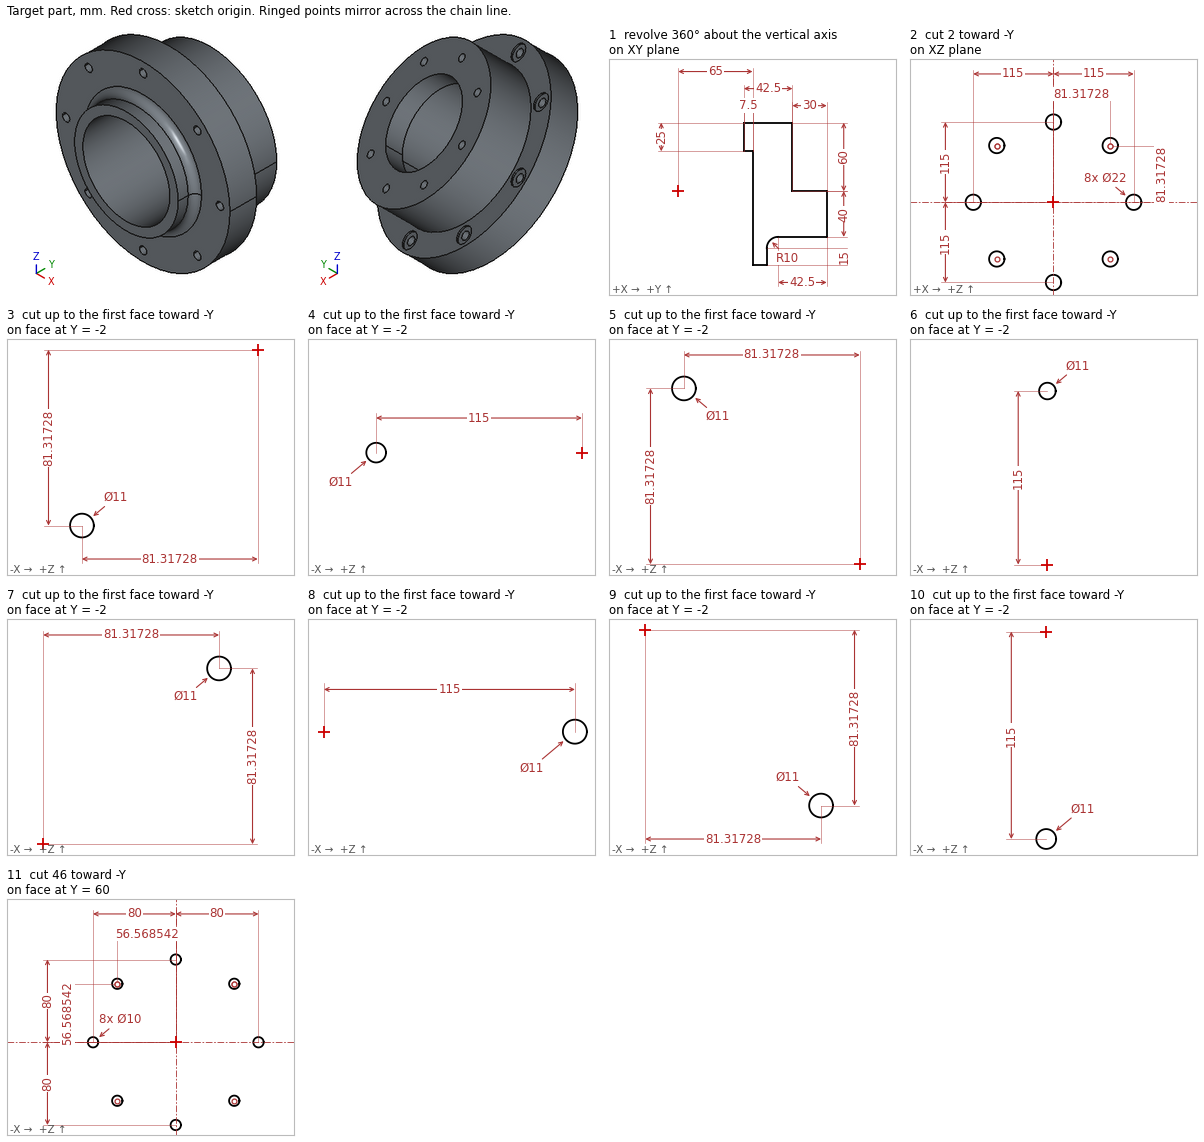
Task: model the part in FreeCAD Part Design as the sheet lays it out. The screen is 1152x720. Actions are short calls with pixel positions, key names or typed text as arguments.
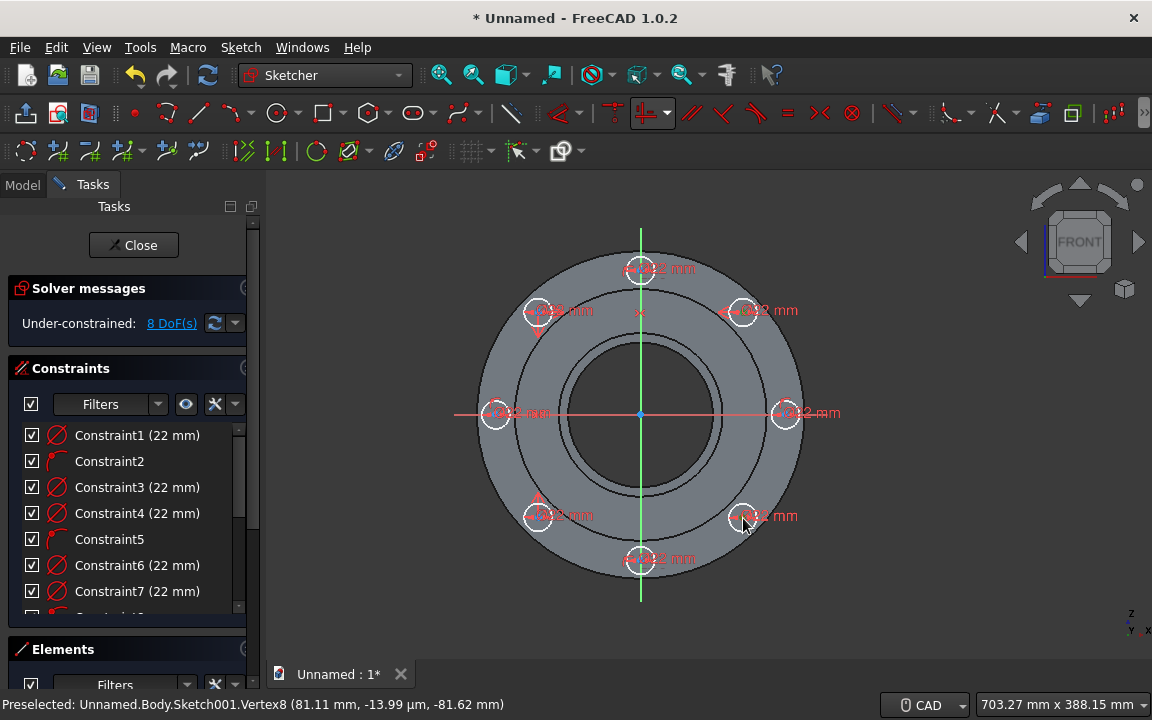
click(591, 415)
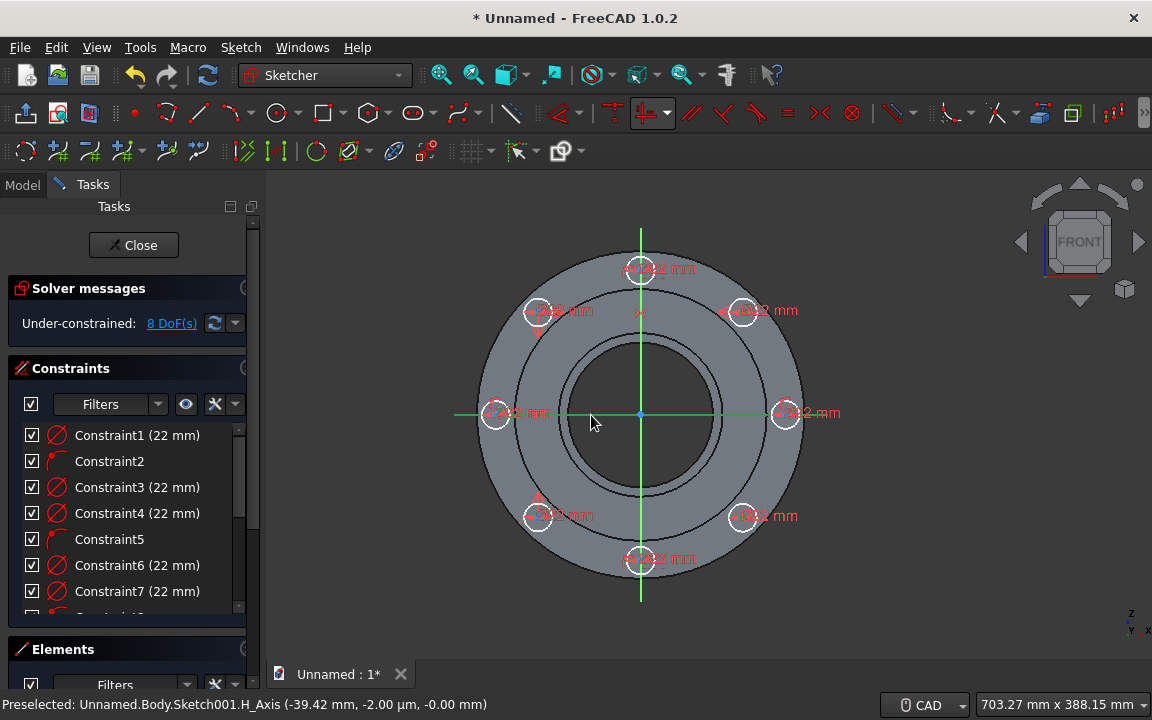
click(820, 114)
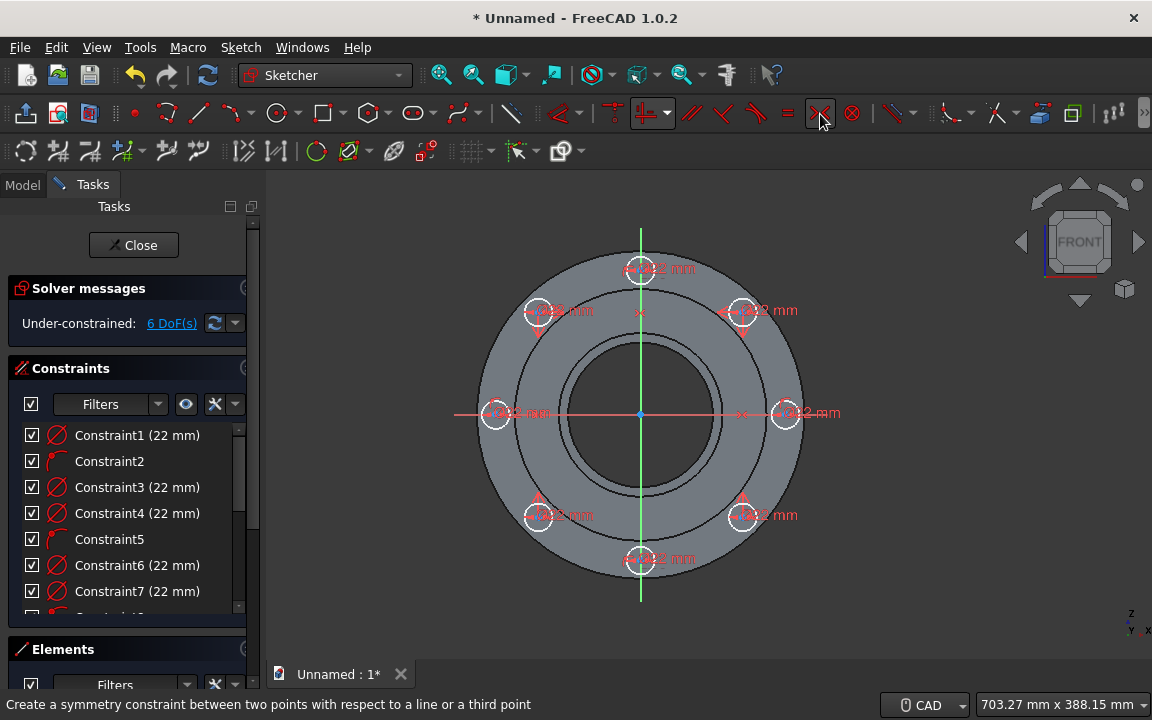
click(558, 114)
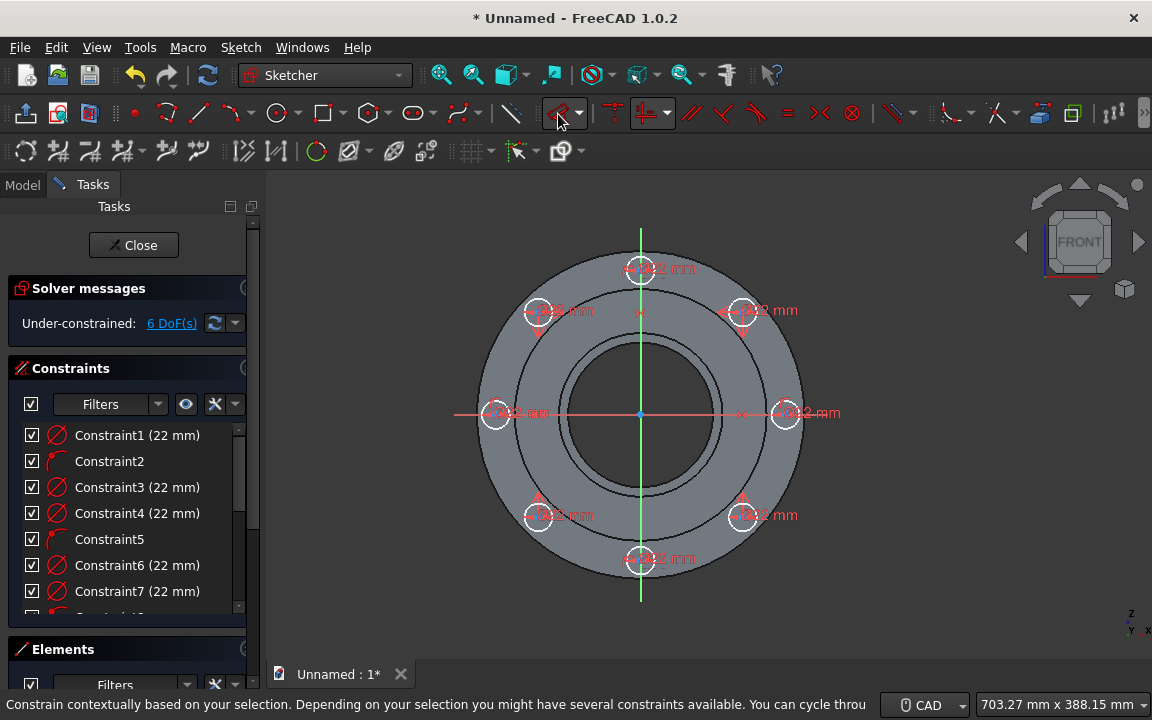
click(786, 415)
click(713, 449)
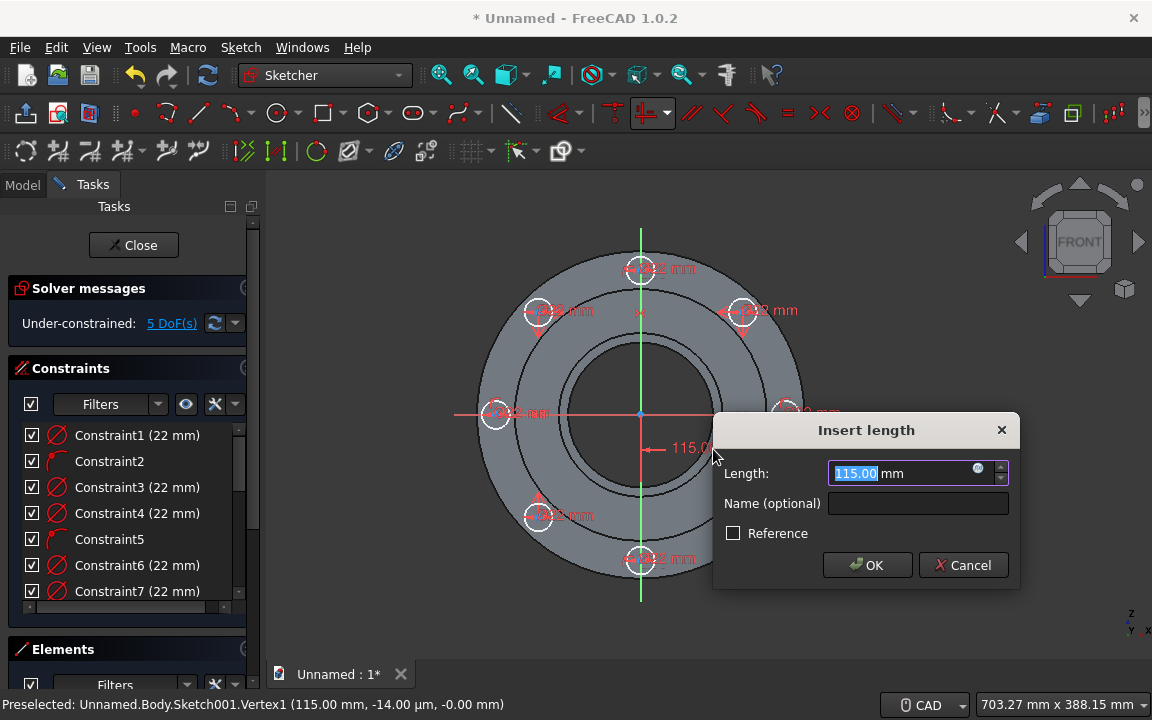
text(115)
key(Return)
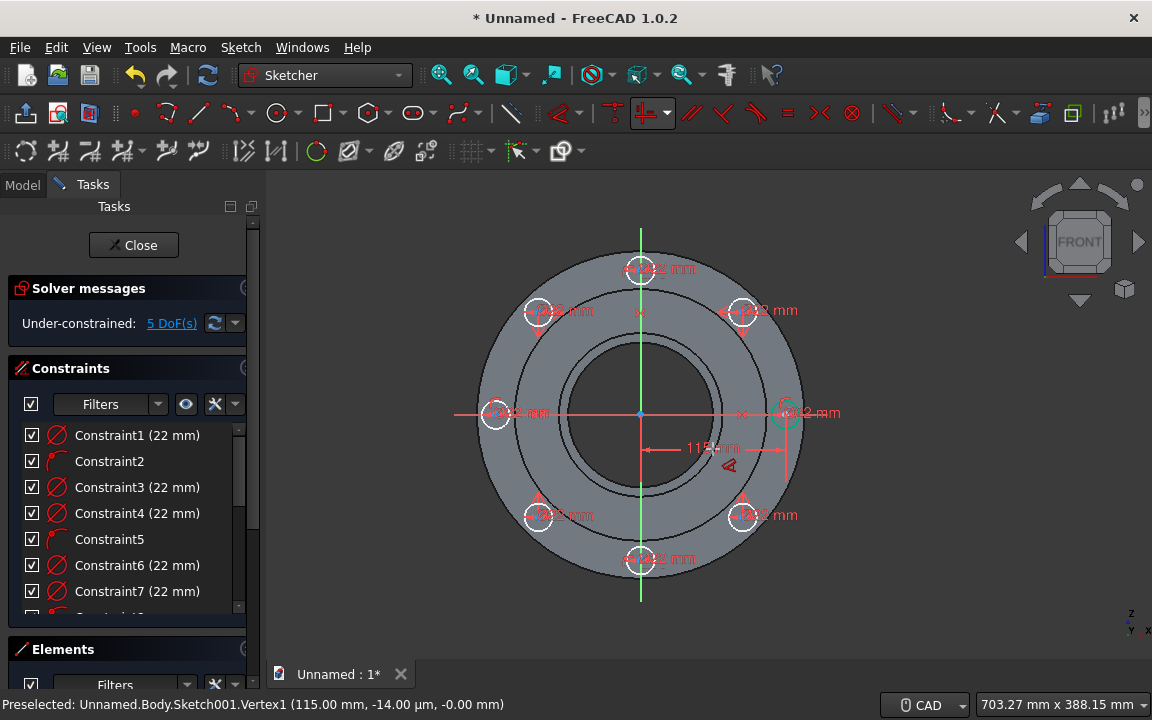
click(641, 271)
click(675, 343)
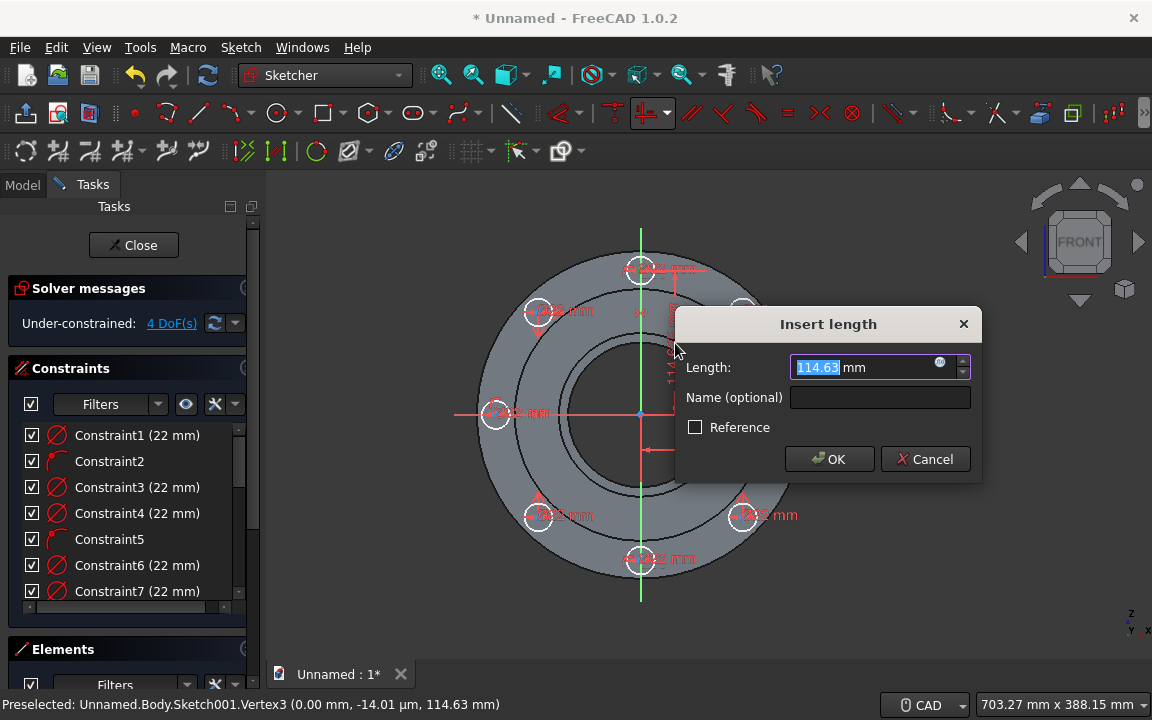
text(115)
key(Return)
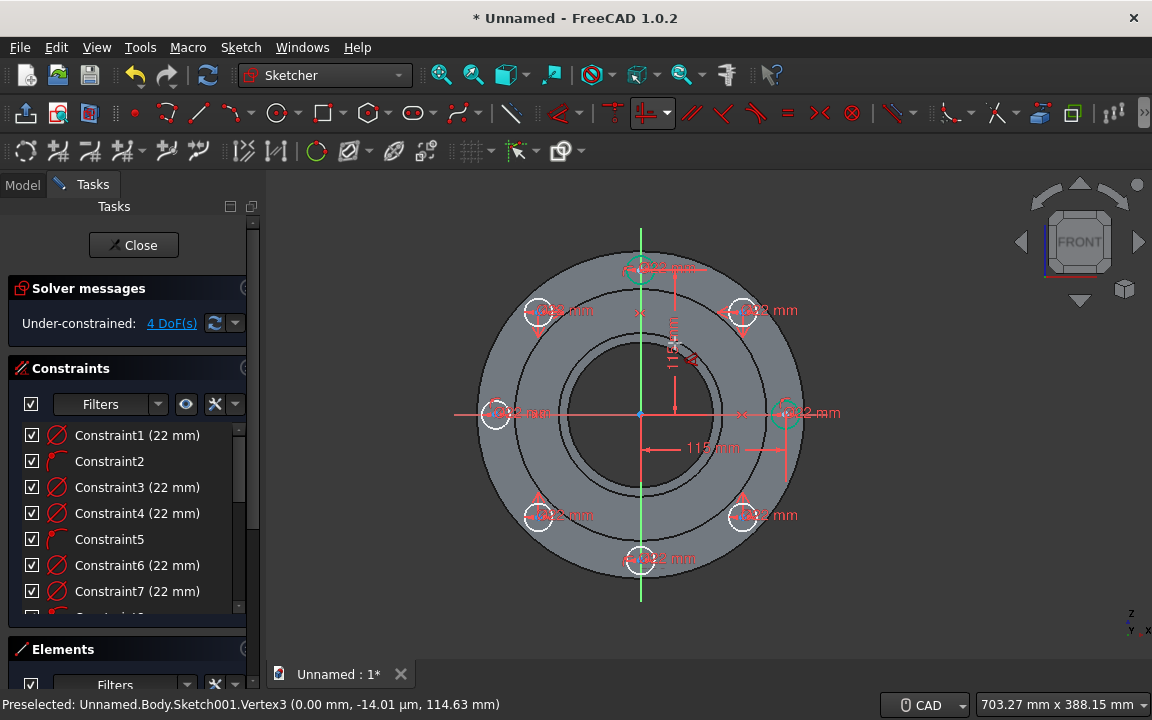
click(496, 415)
click(568, 449)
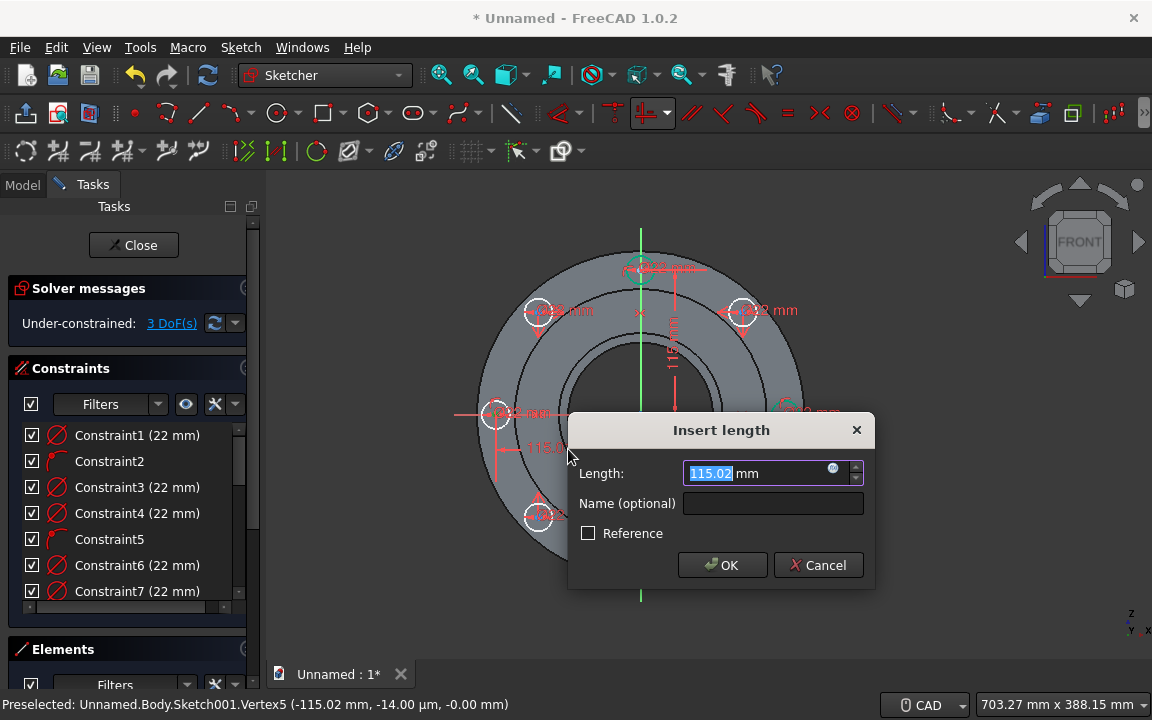
text(115)
key(Return)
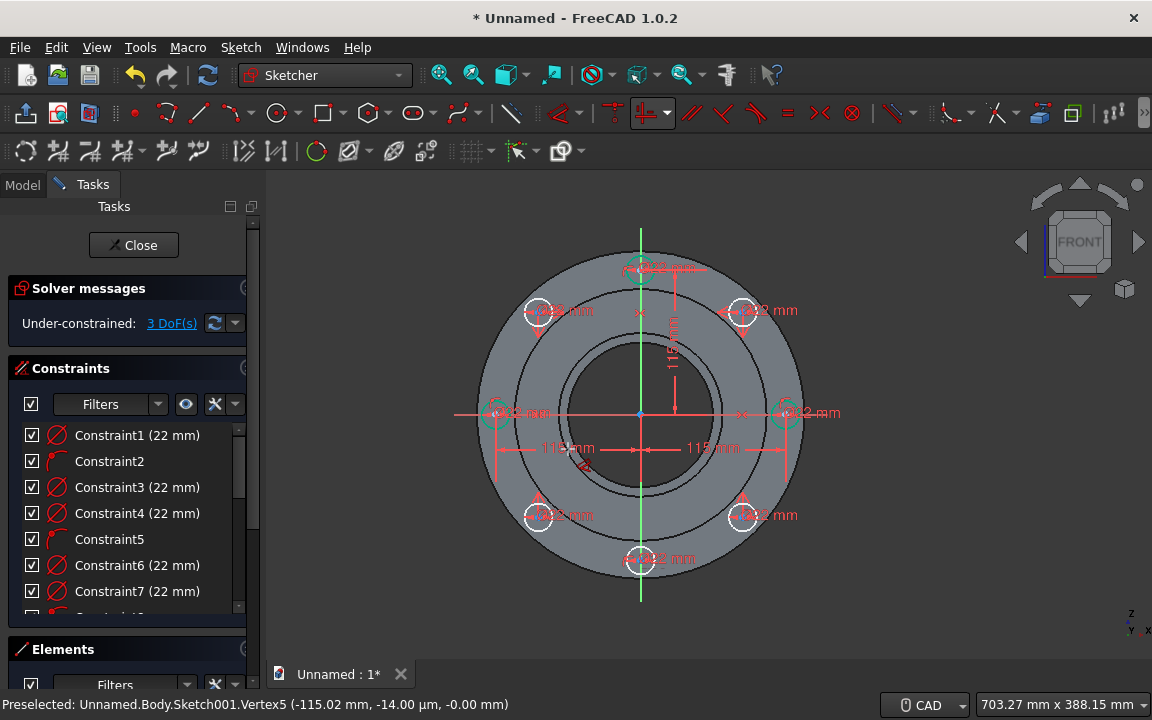
click(641, 561)
click(675, 488)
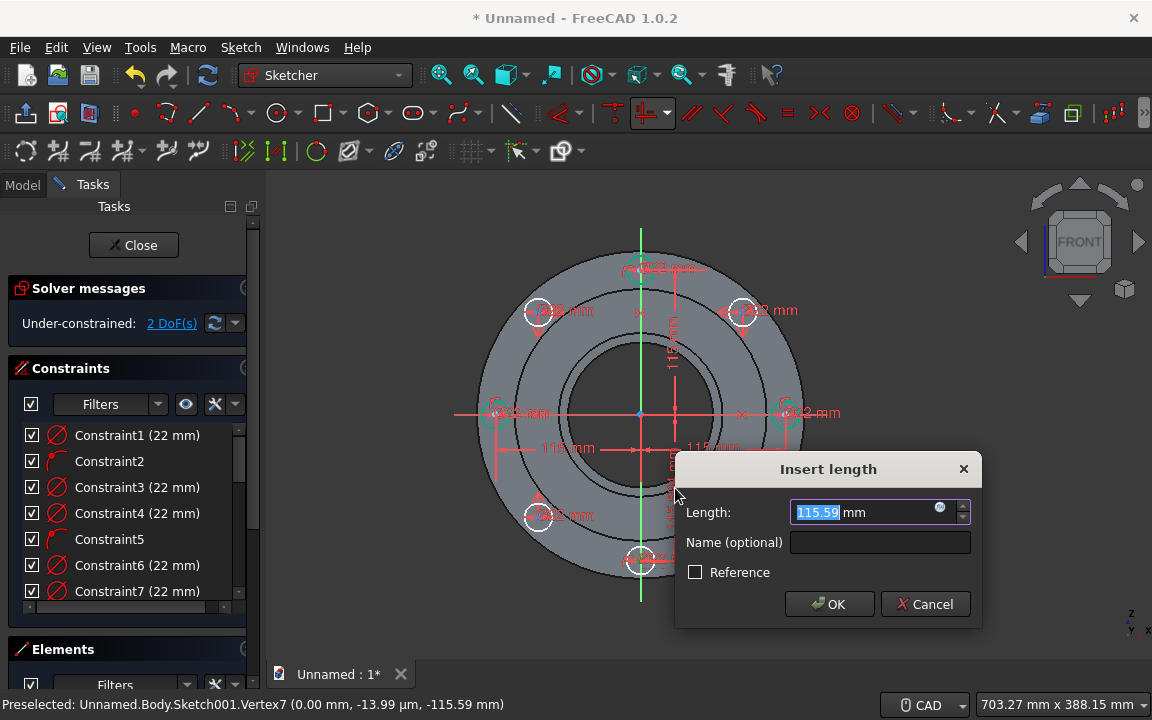
text(115)
key(Return)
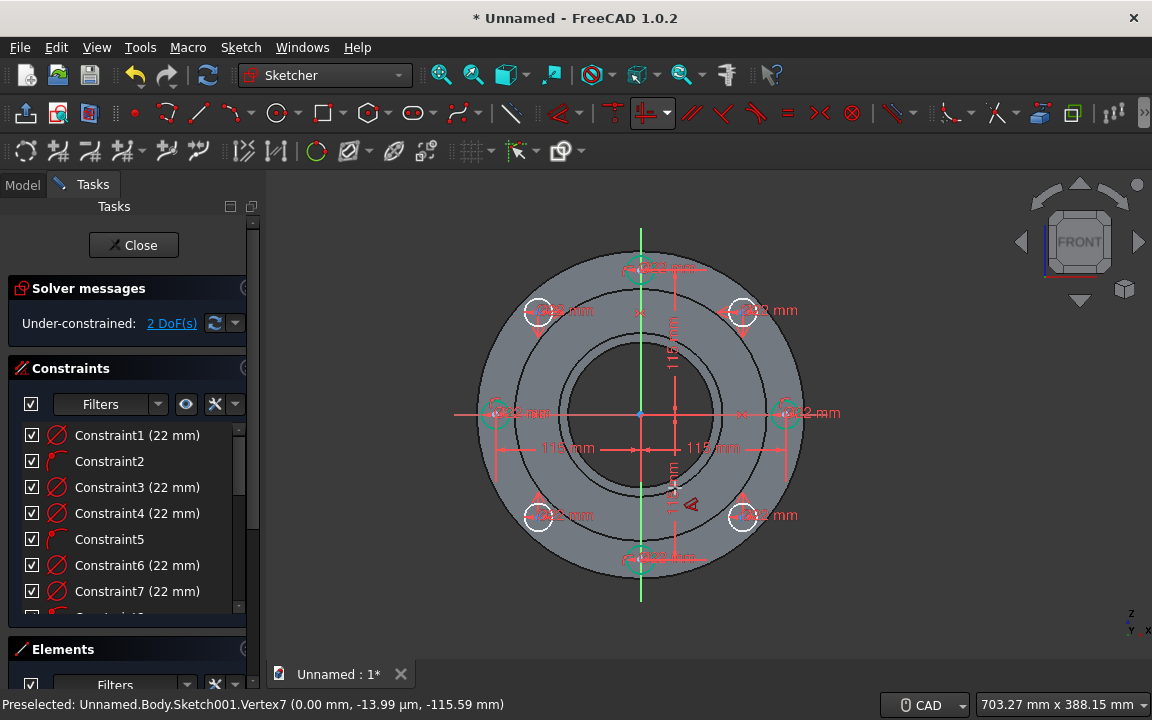
click(743, 312)
click(692, 278)